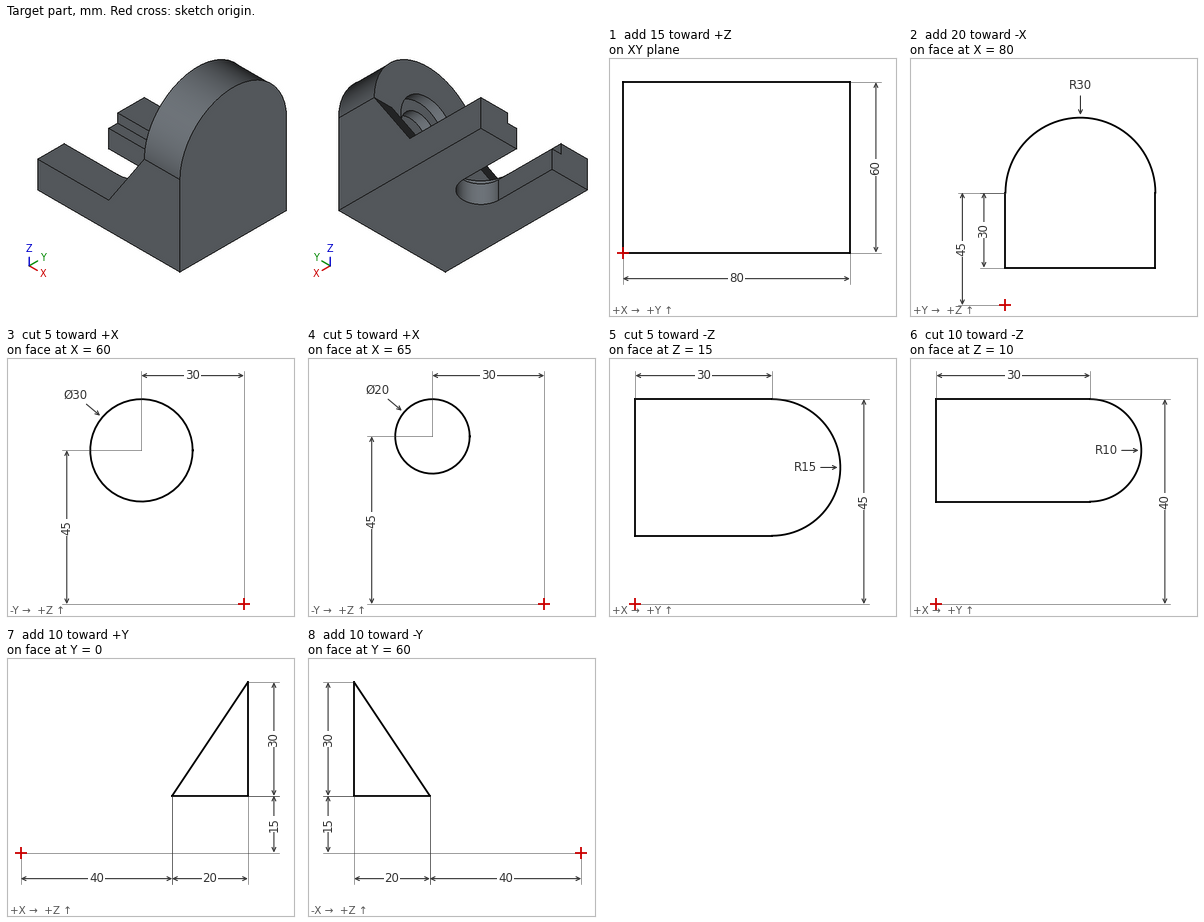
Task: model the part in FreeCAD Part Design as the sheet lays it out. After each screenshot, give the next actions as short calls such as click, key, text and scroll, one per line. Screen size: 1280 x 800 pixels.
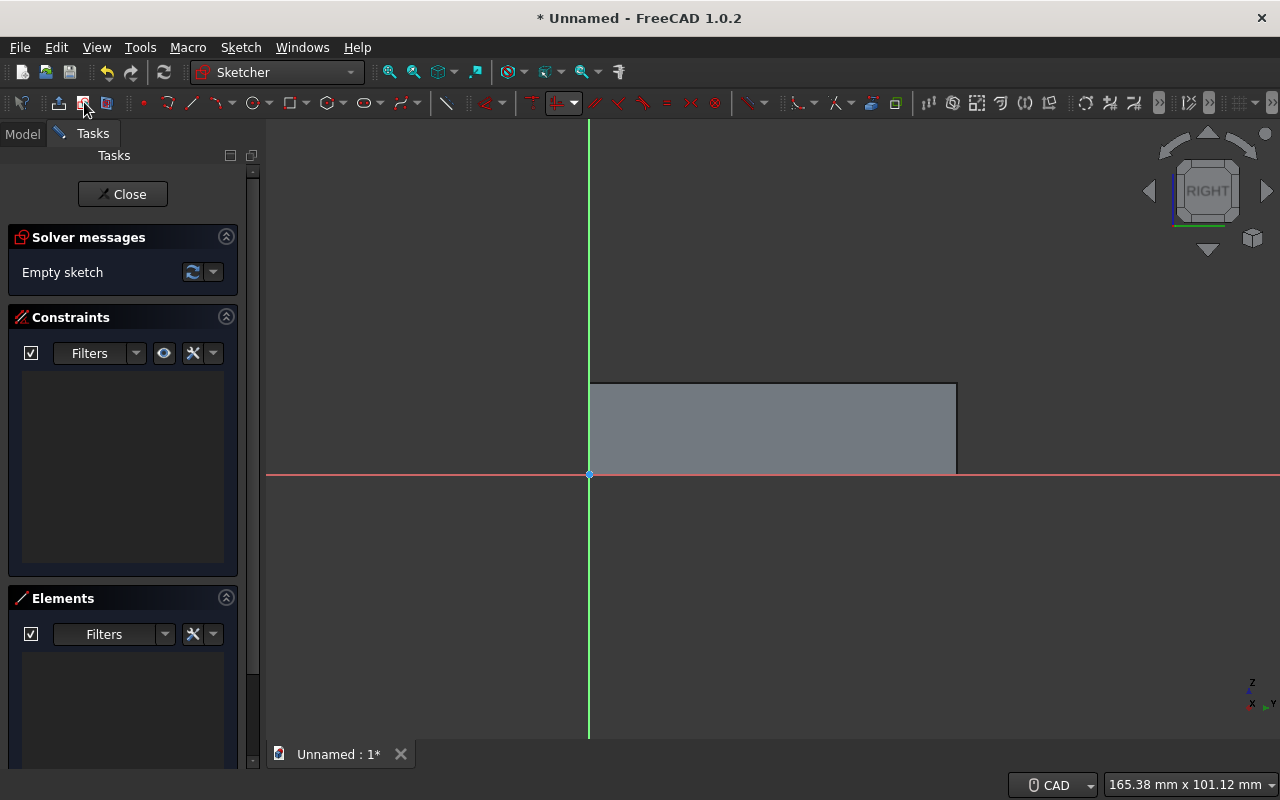
scroll(565, 711, down, 2)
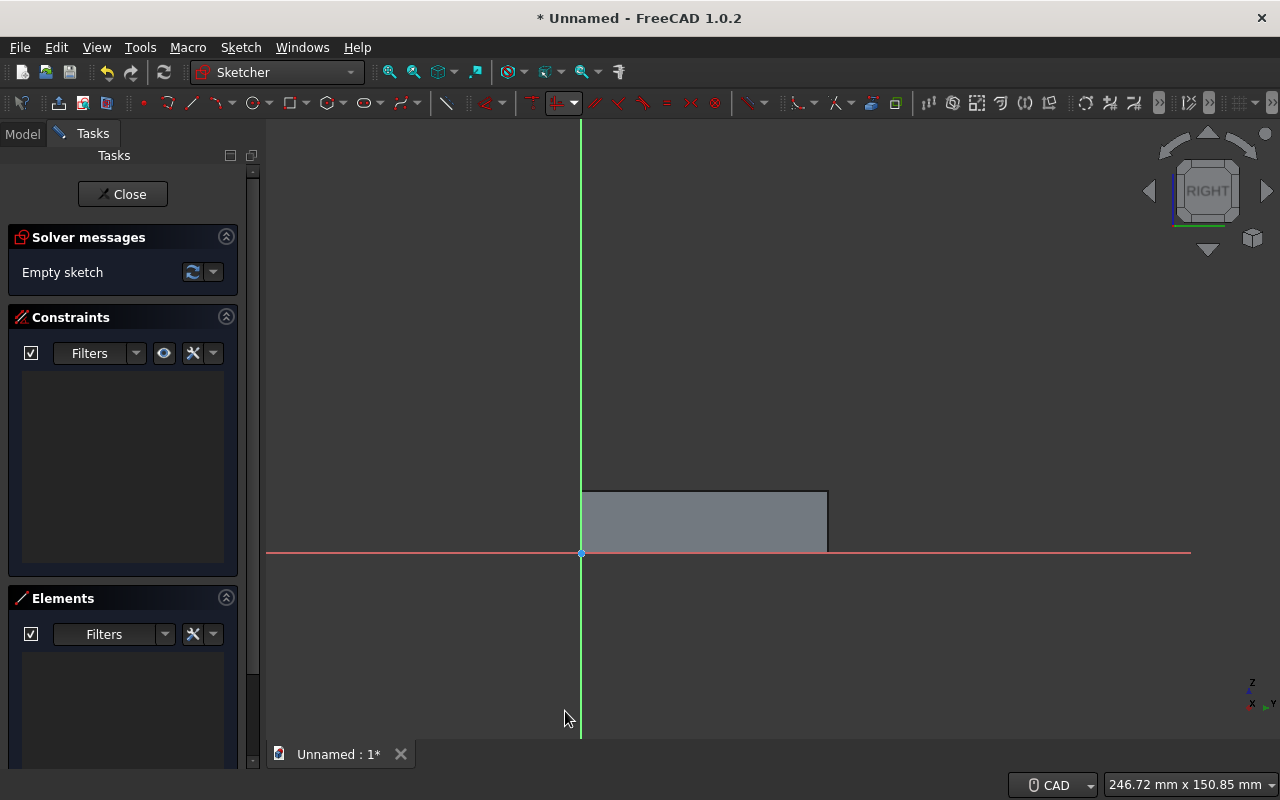
click(168, 104)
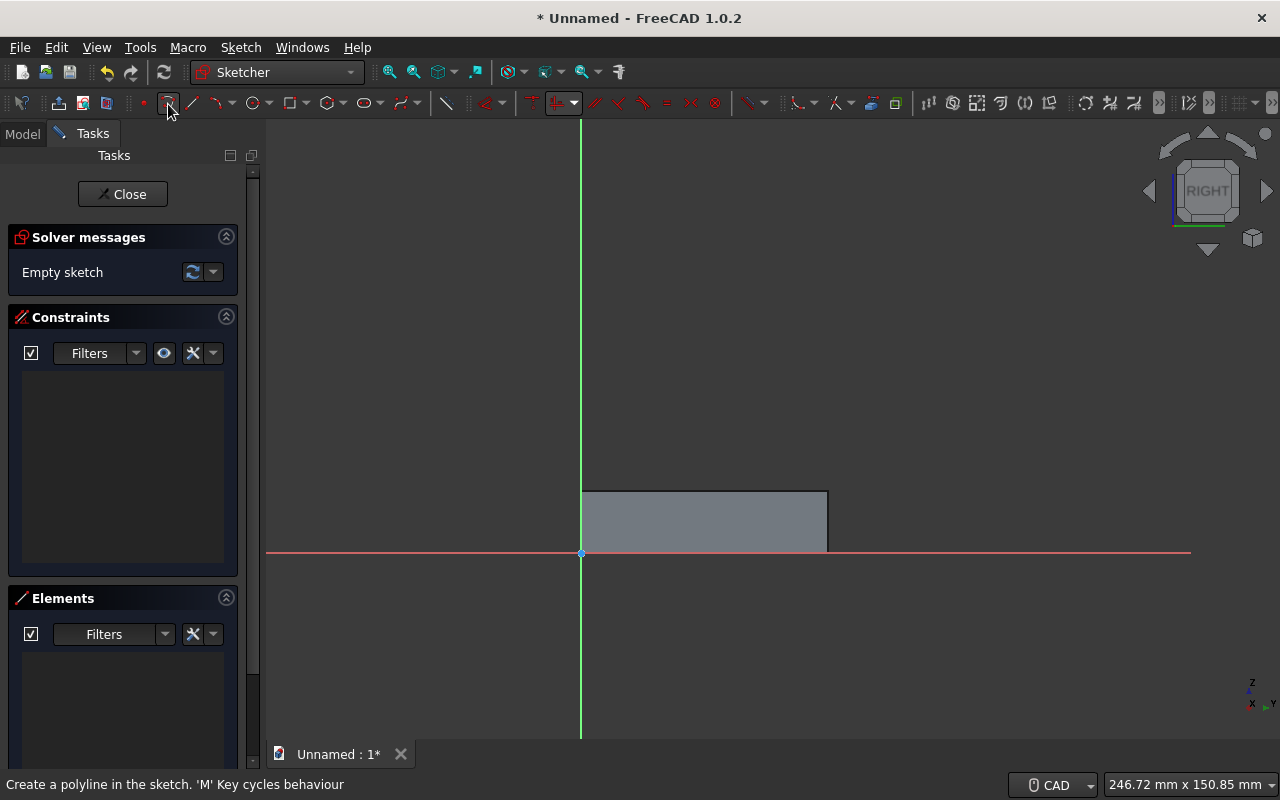
click(581, 368)
click(590, 491)
click(828, 491)
click(828, 368)
right_click(828, 368)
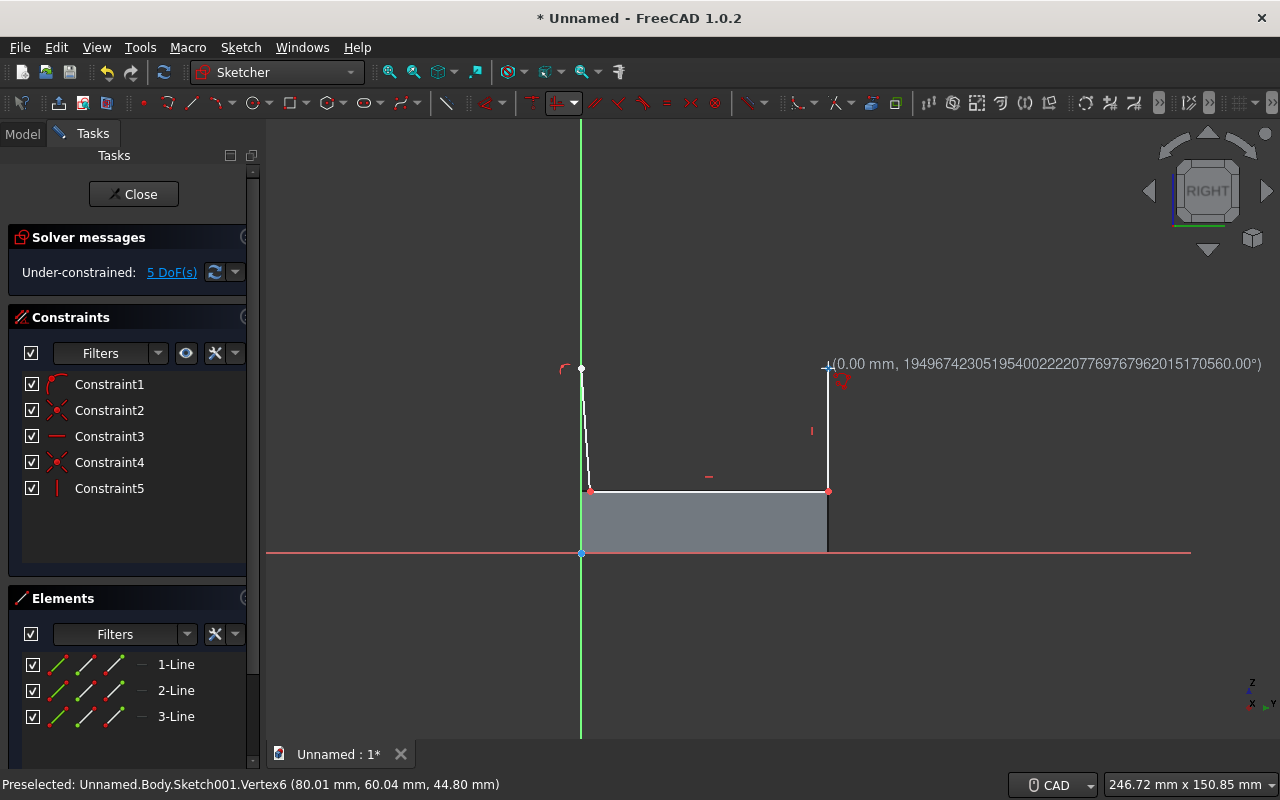
click(216, 104)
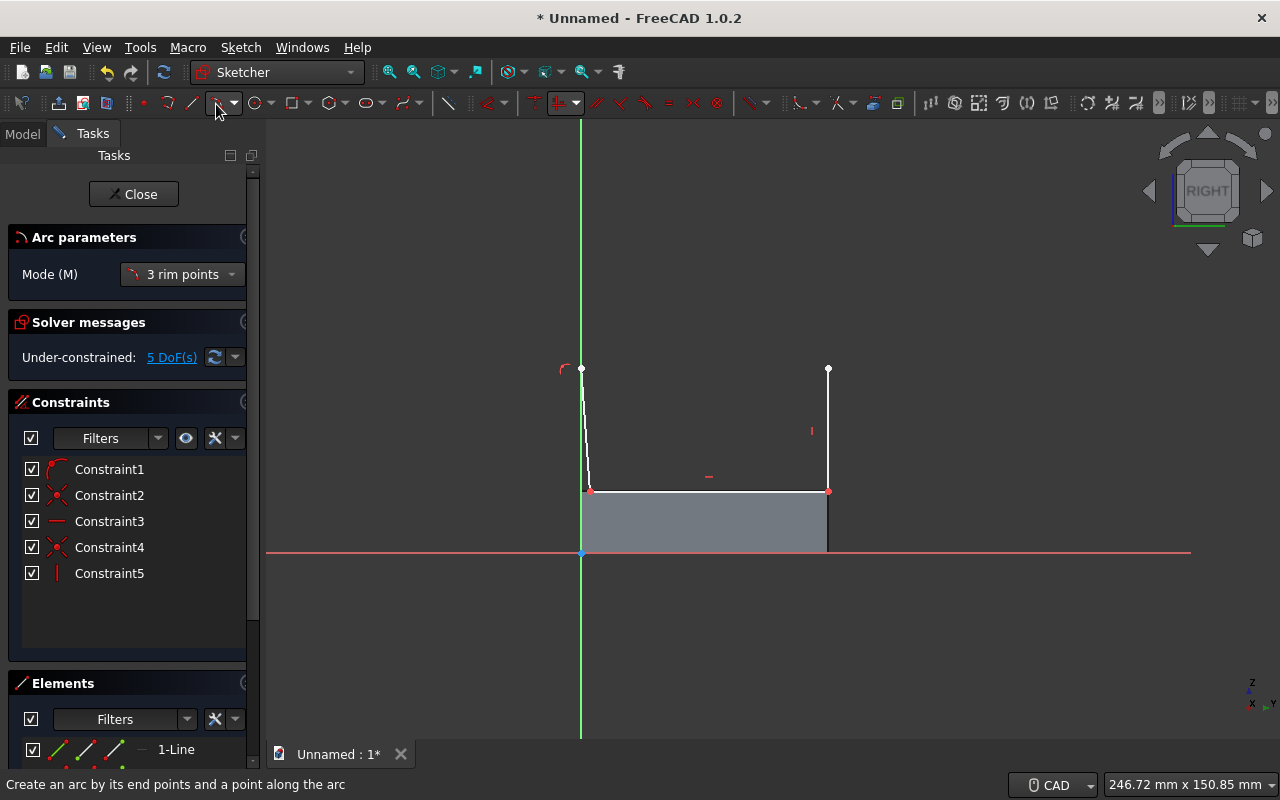
click(828, 369)
click(581, 369)
click(705, 245)
key(Escape)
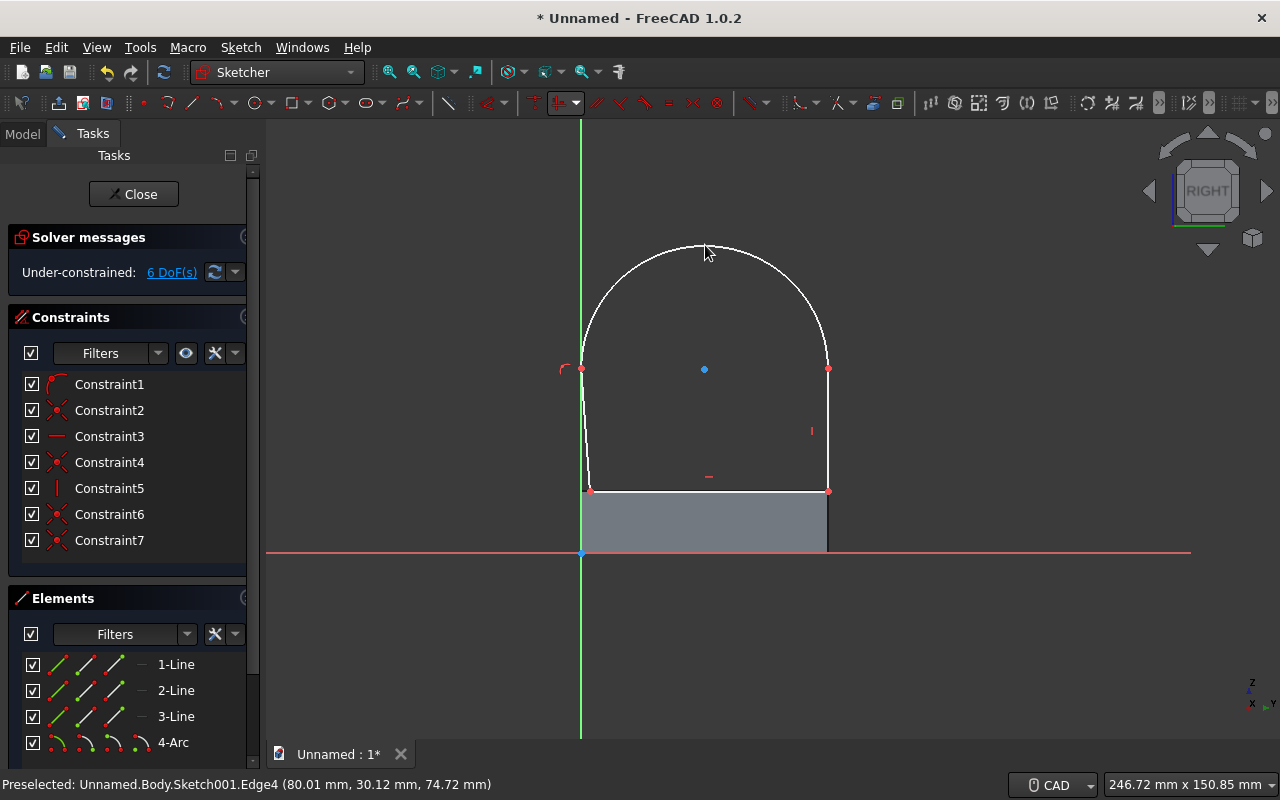
click(584, 406)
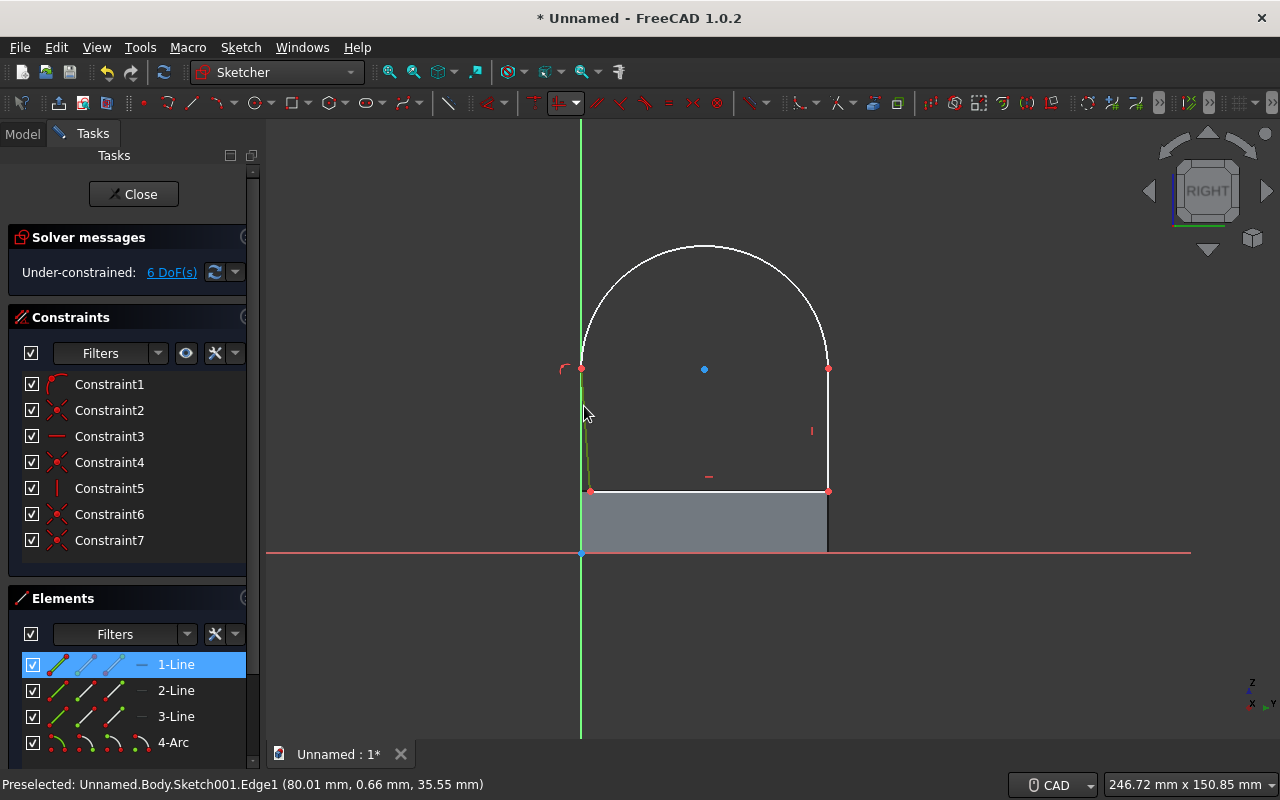
click(777, 269)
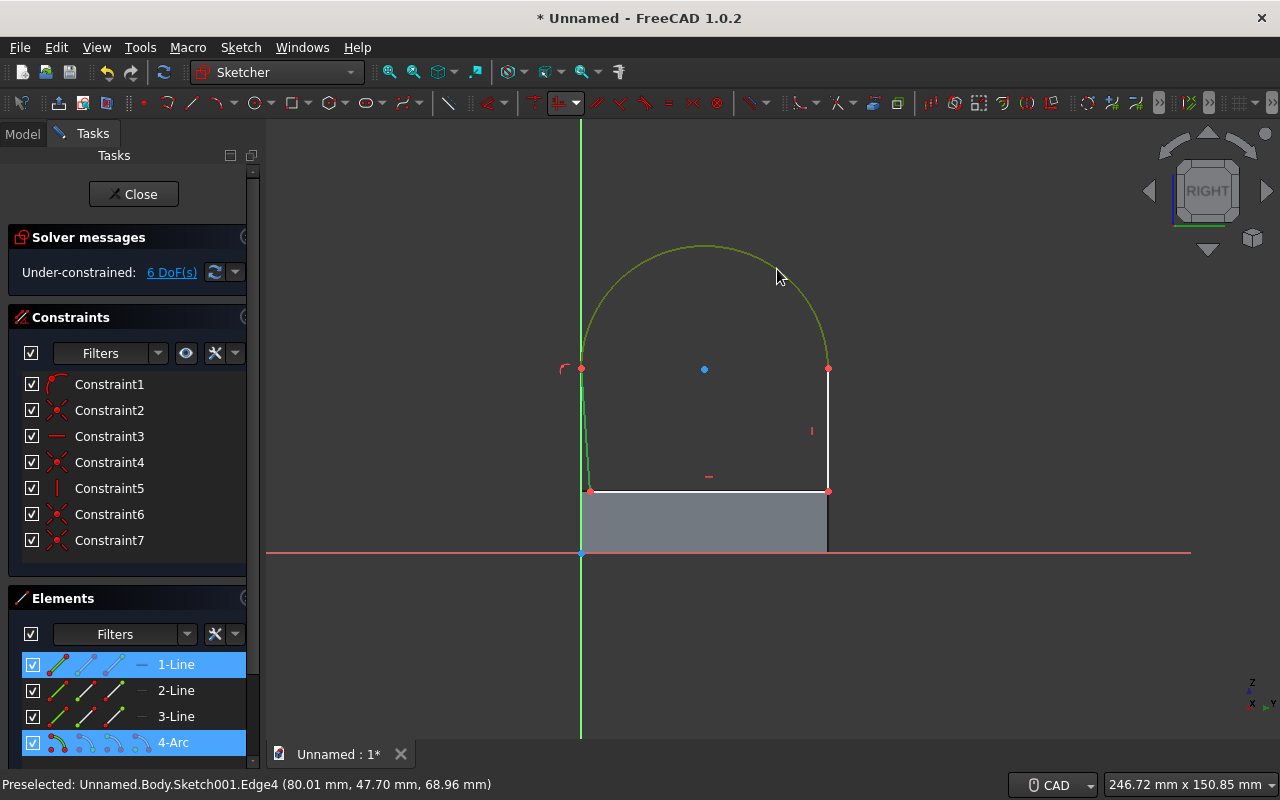
click(646, 104)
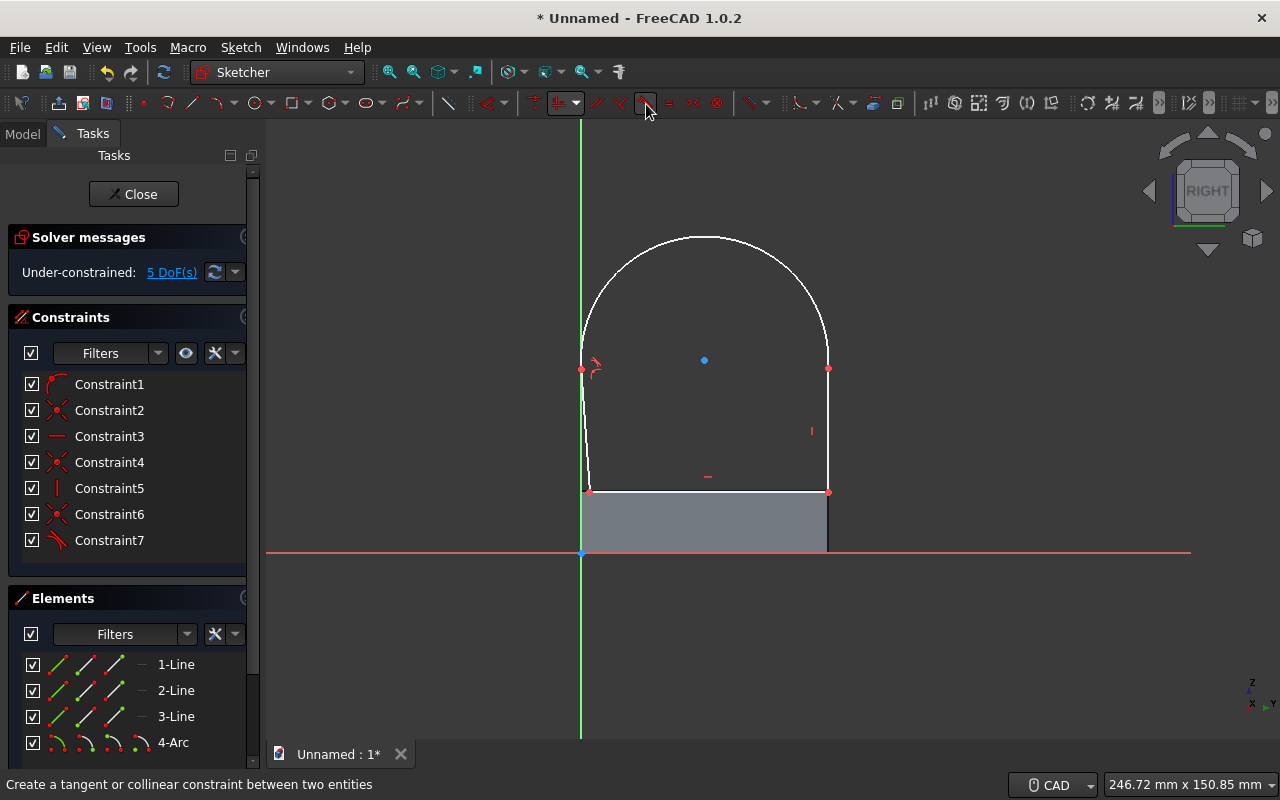
click(828, 455)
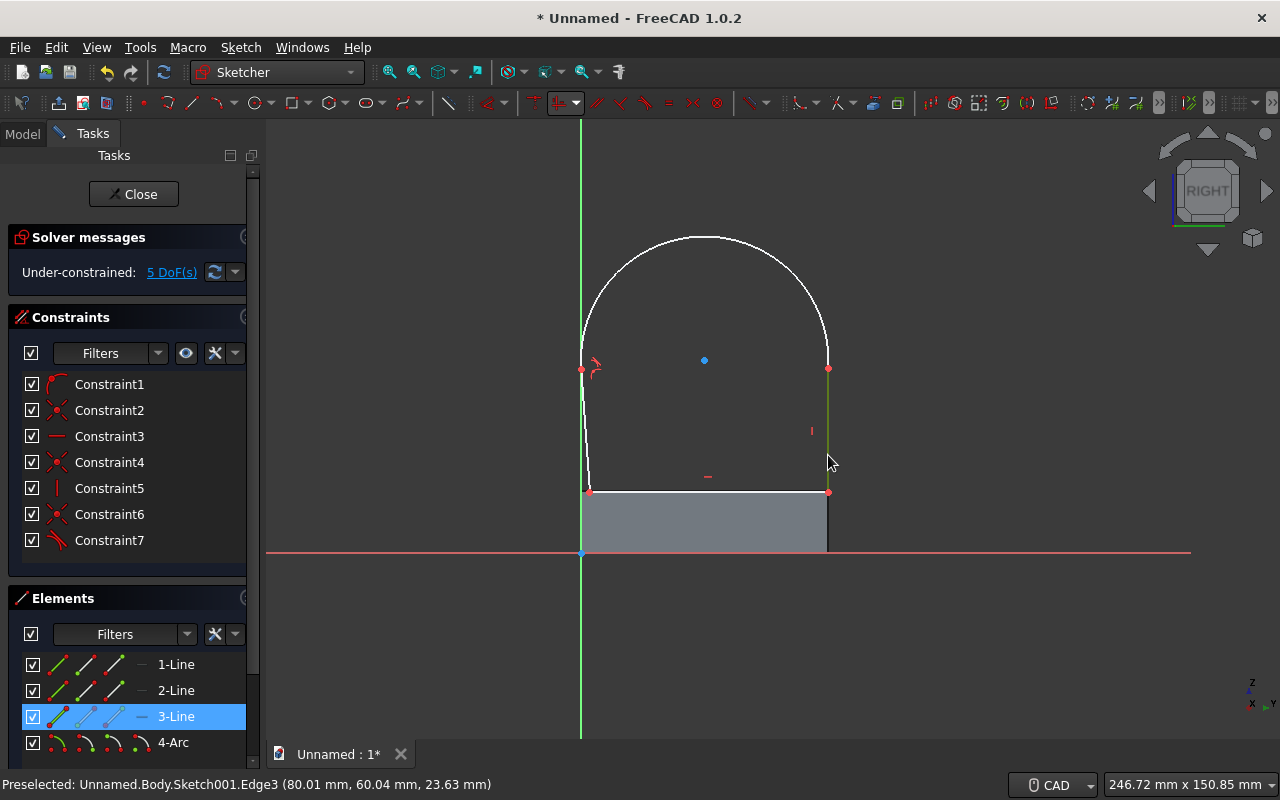
click(780, 262)